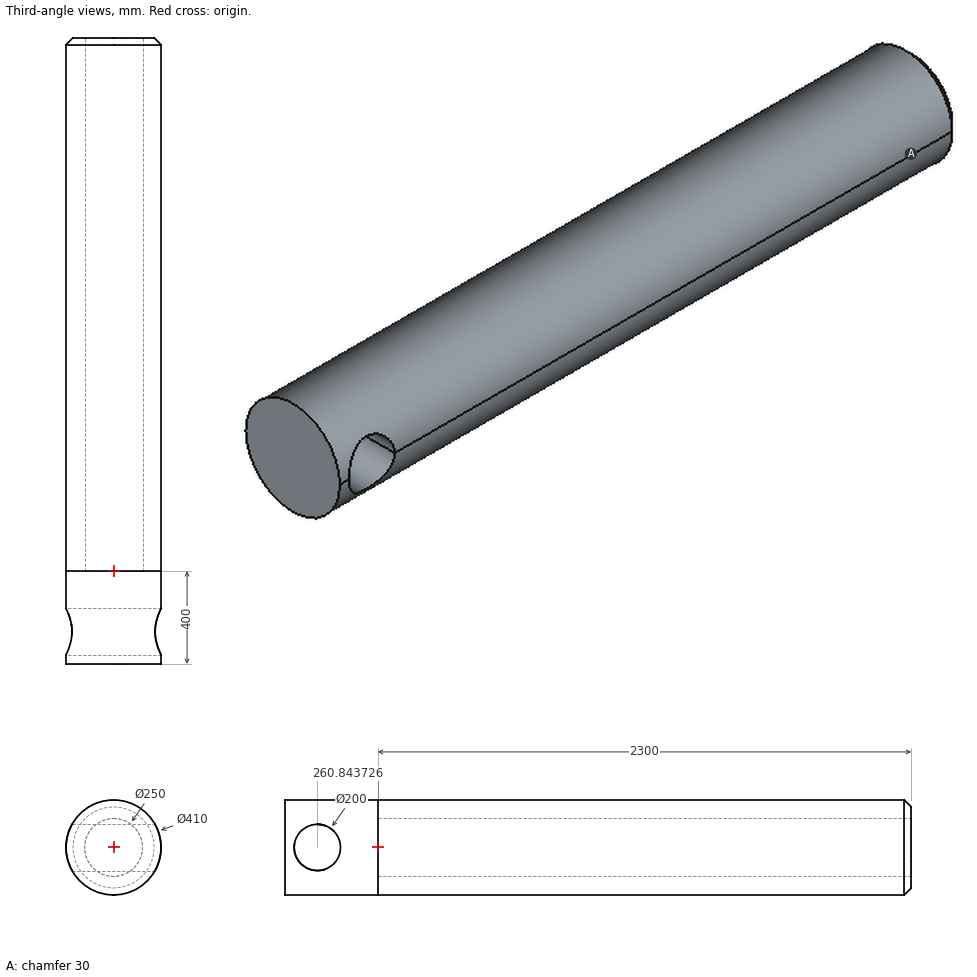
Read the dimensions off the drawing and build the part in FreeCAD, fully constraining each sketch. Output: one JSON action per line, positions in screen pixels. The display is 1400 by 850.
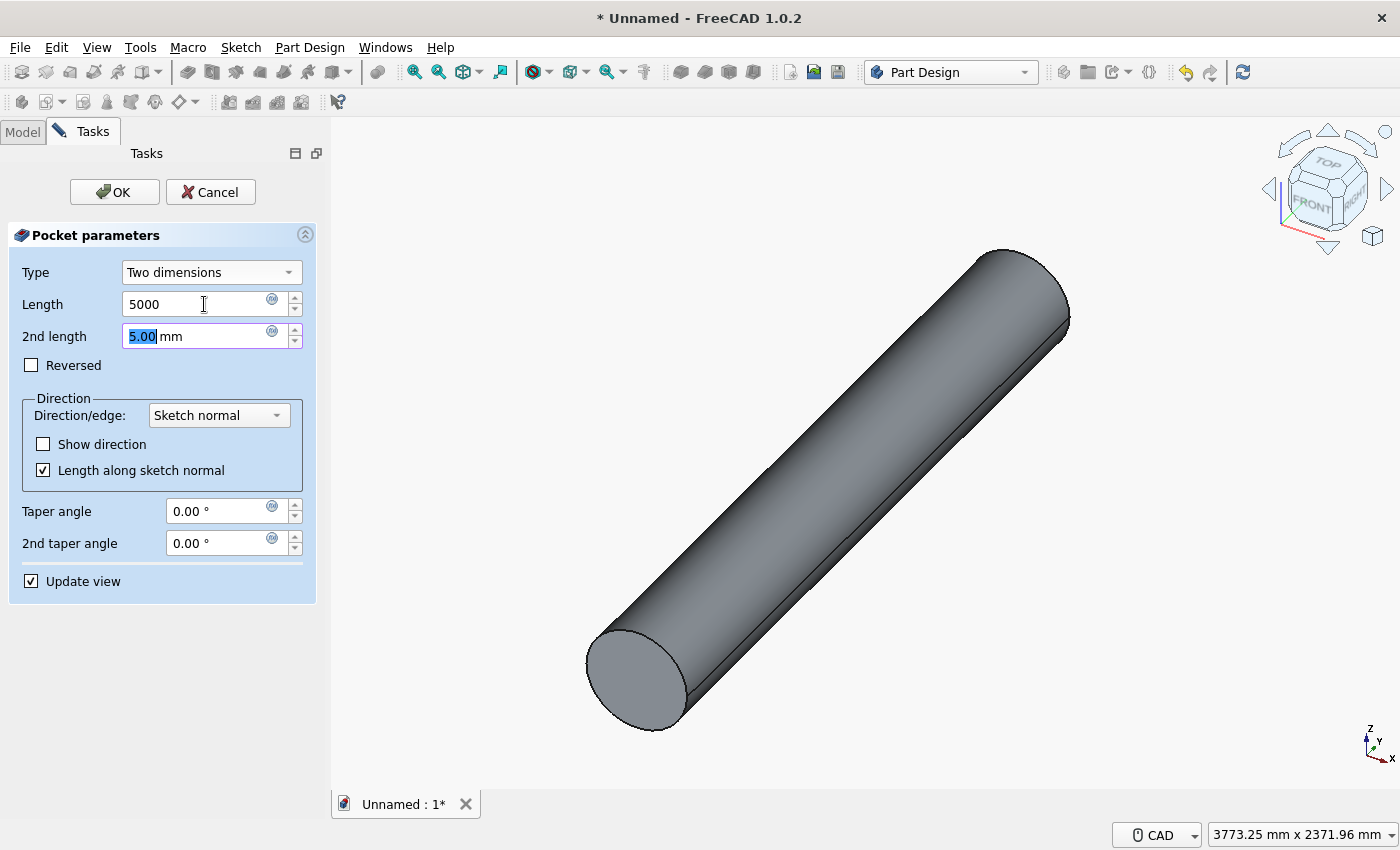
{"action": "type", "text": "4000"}
{"action": "key", "text": "Tab"}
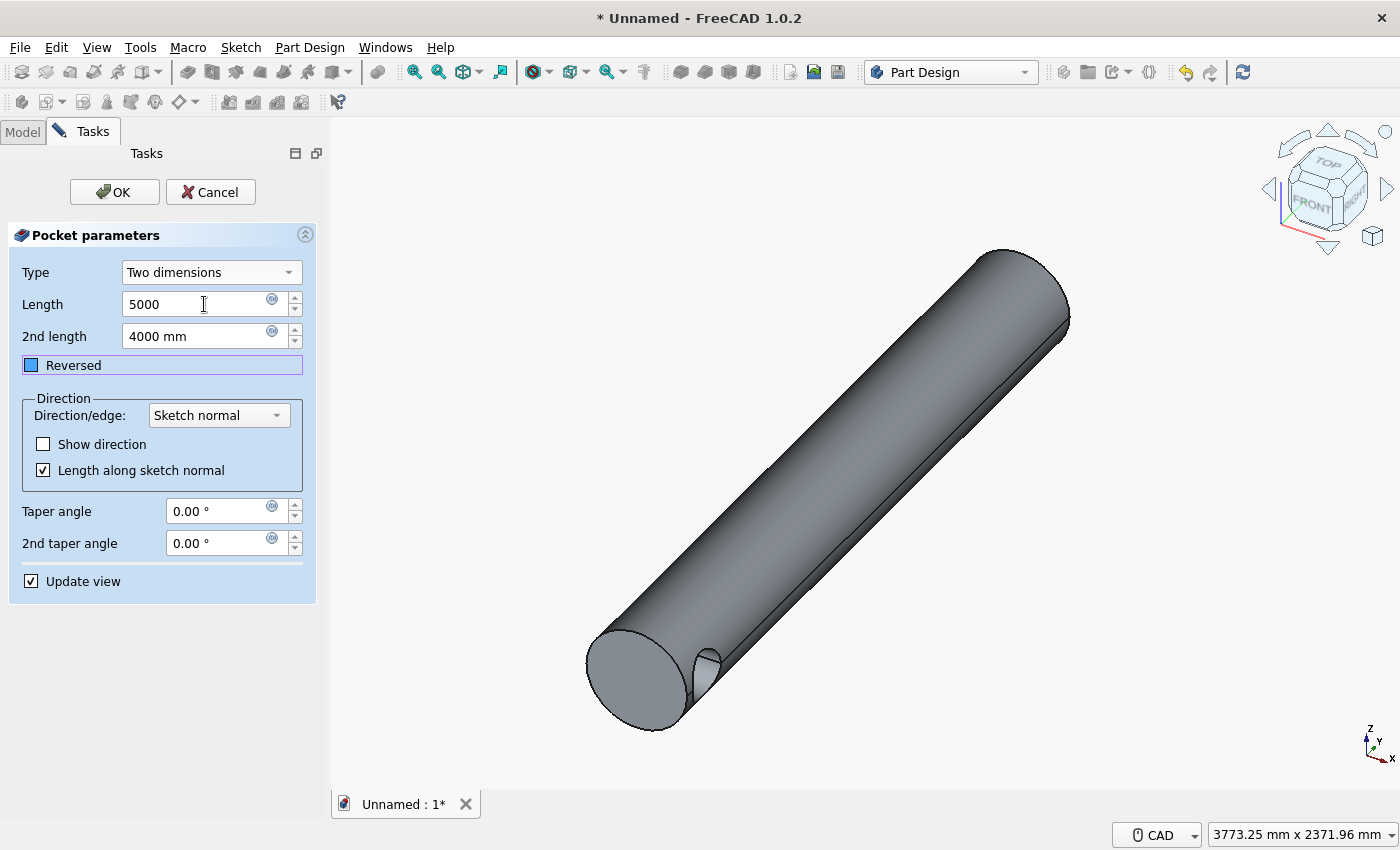
{"action": "left_click", "coordinate": [30, 365]}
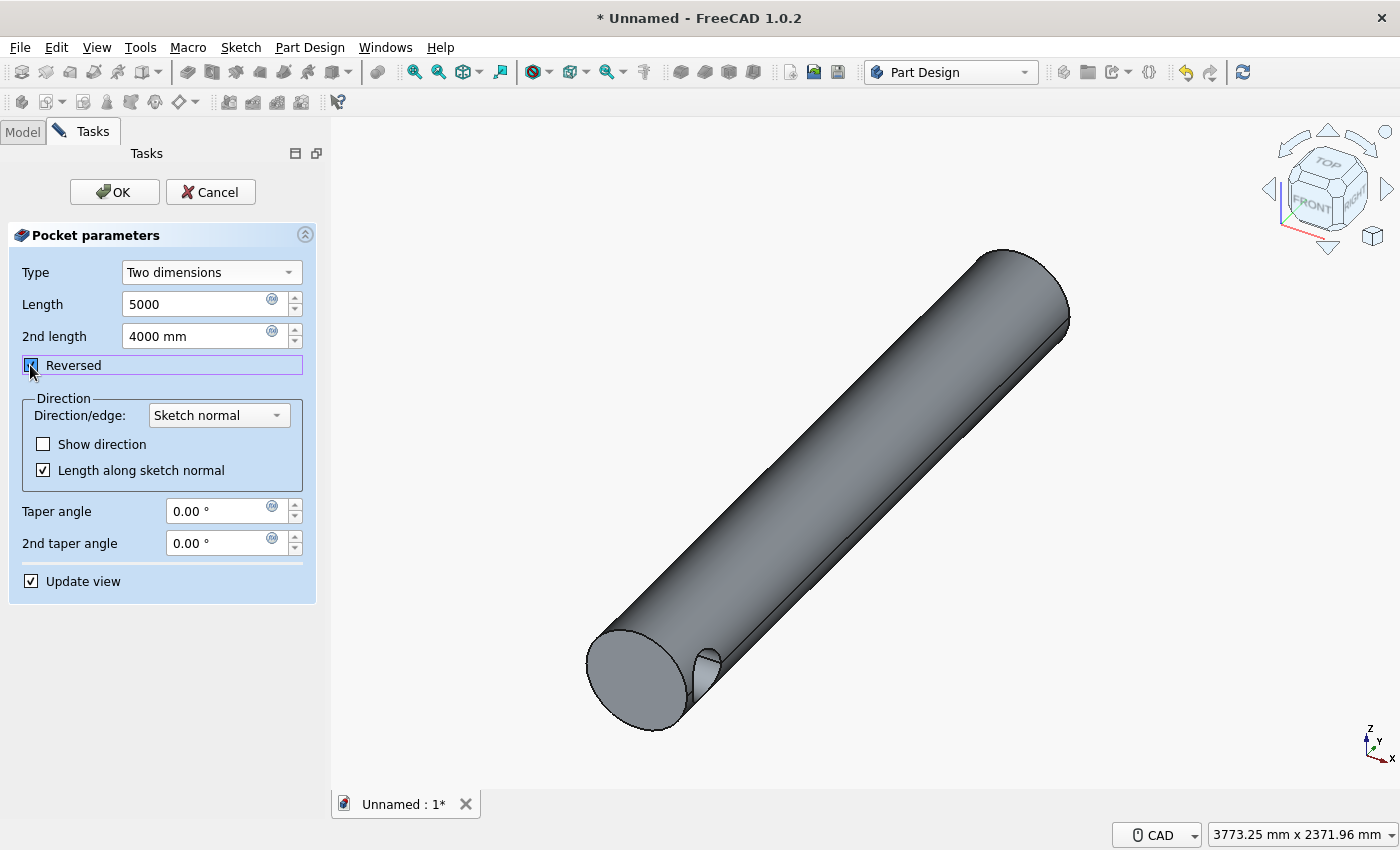
{"action": "left_click", "coordinate": [115, 192]}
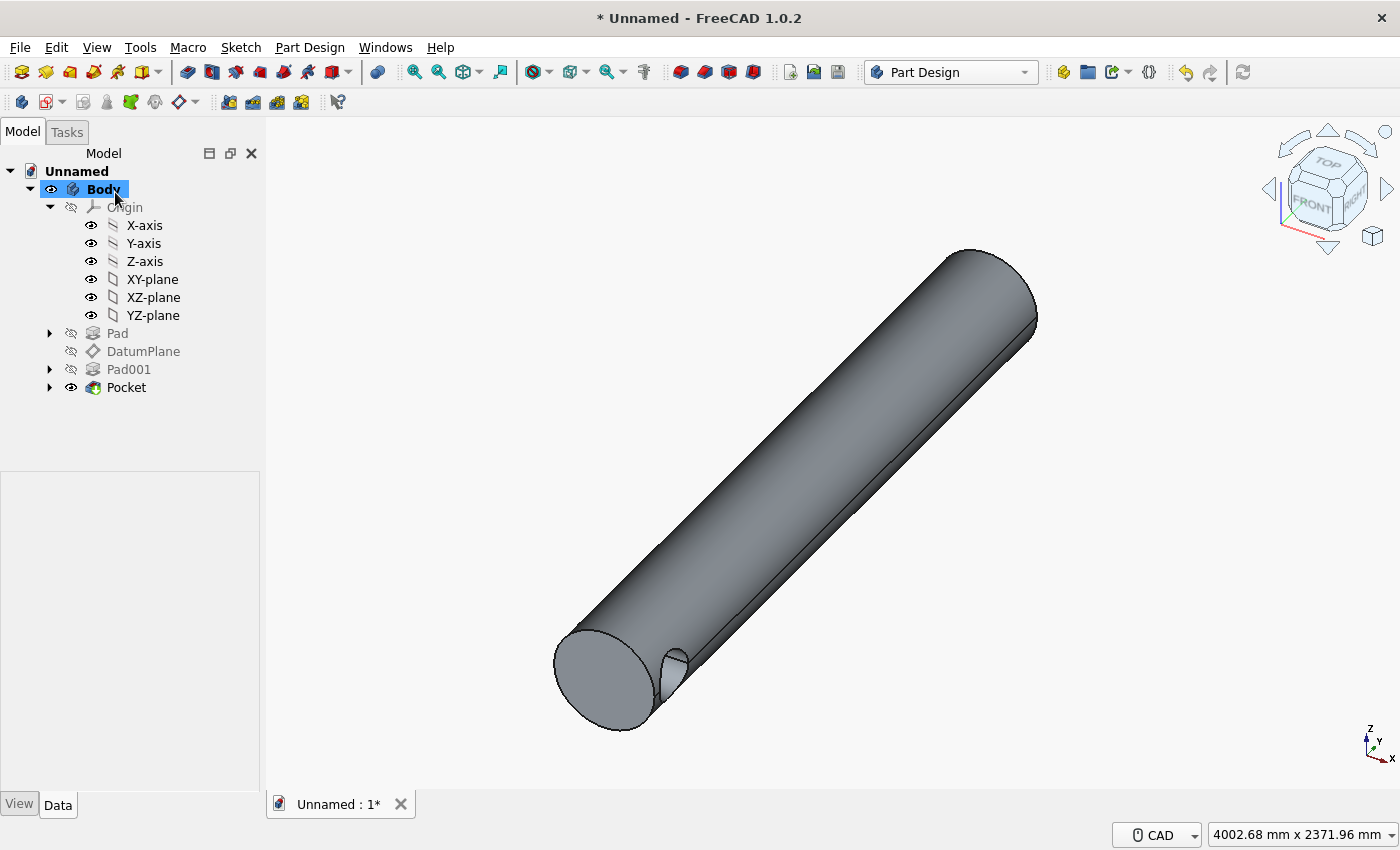
{"action": "key", "text": "0"}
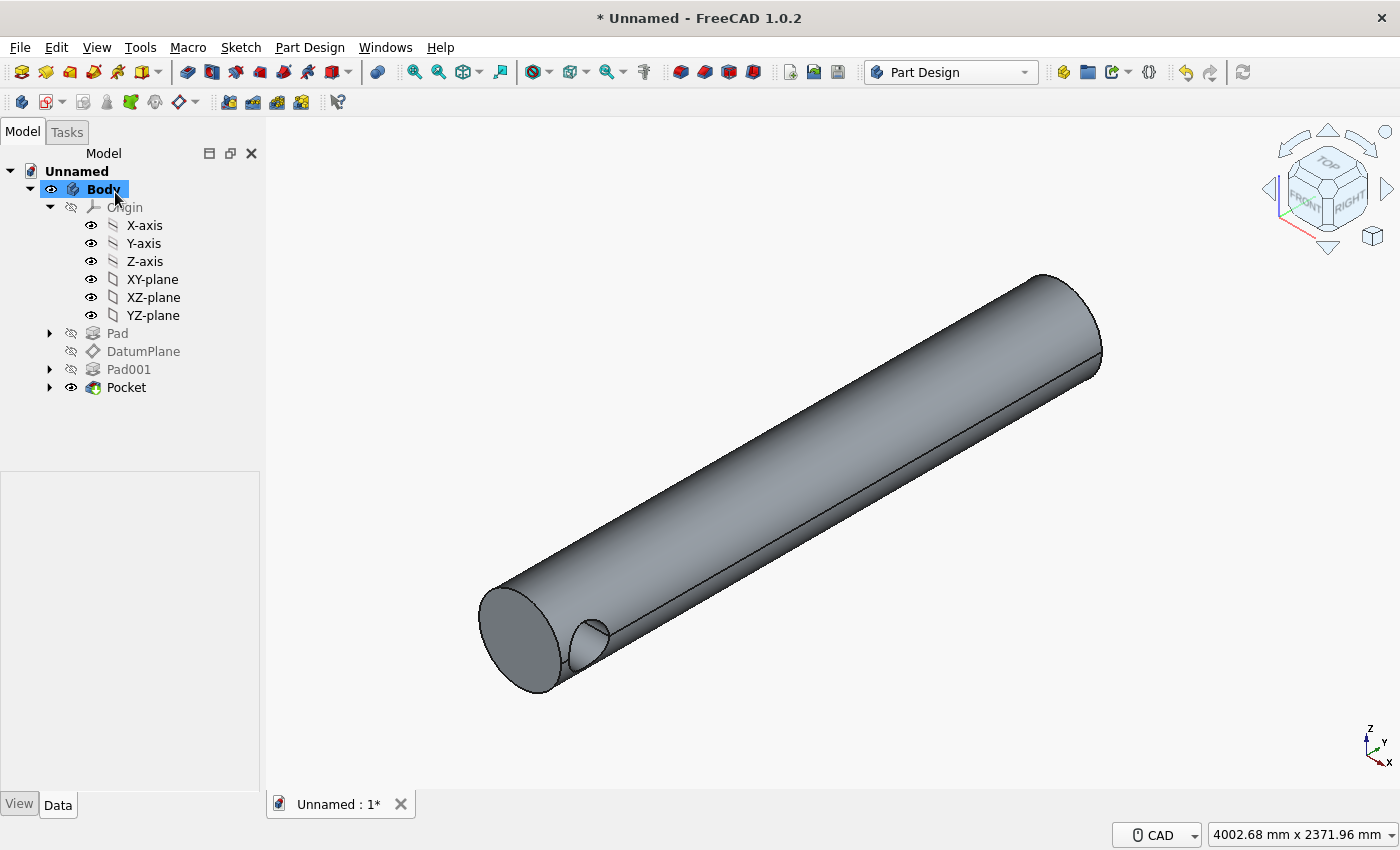
{"action": "key", "text": "2"}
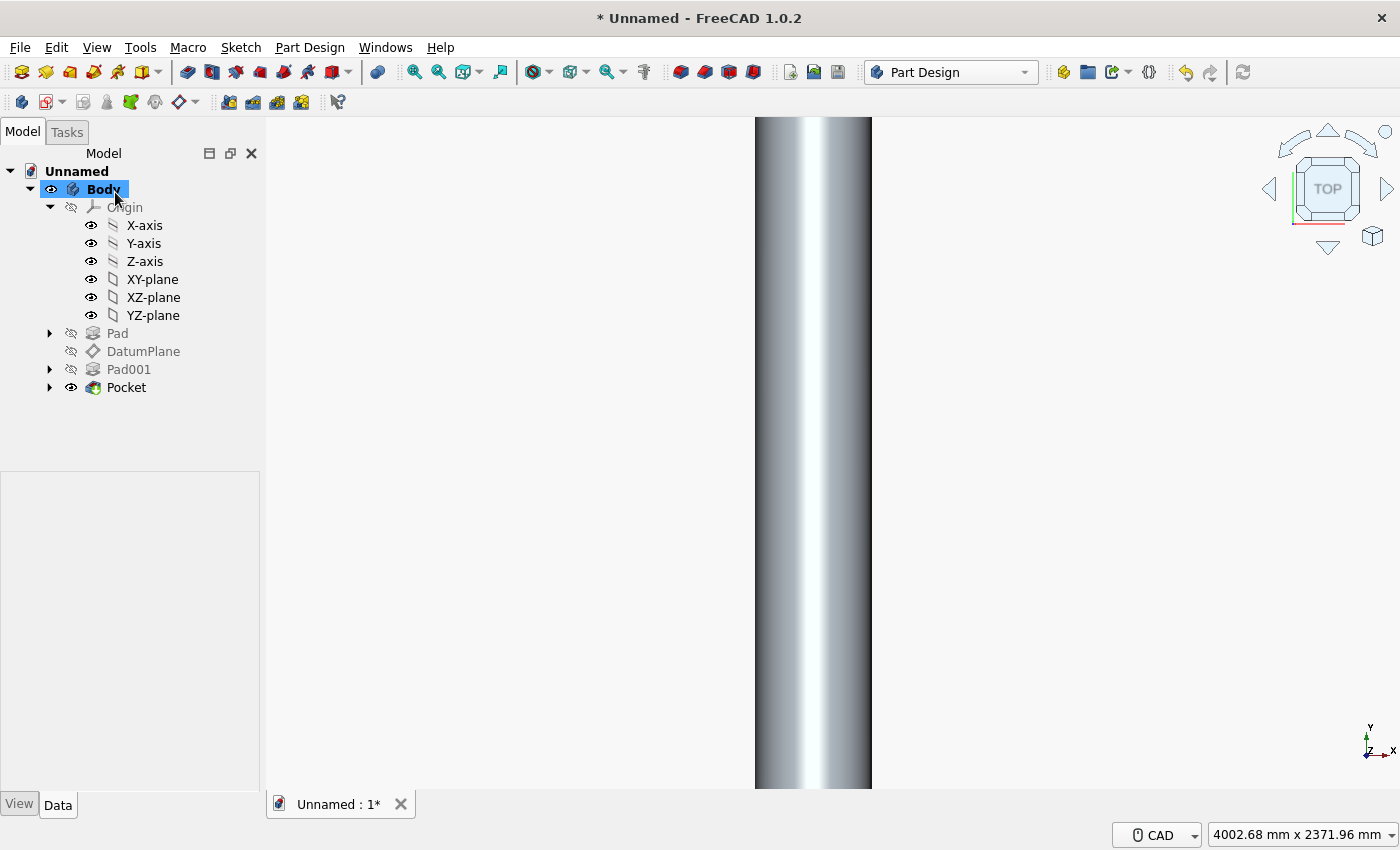
{"action": "left_click", "coordinate": [416, 72]}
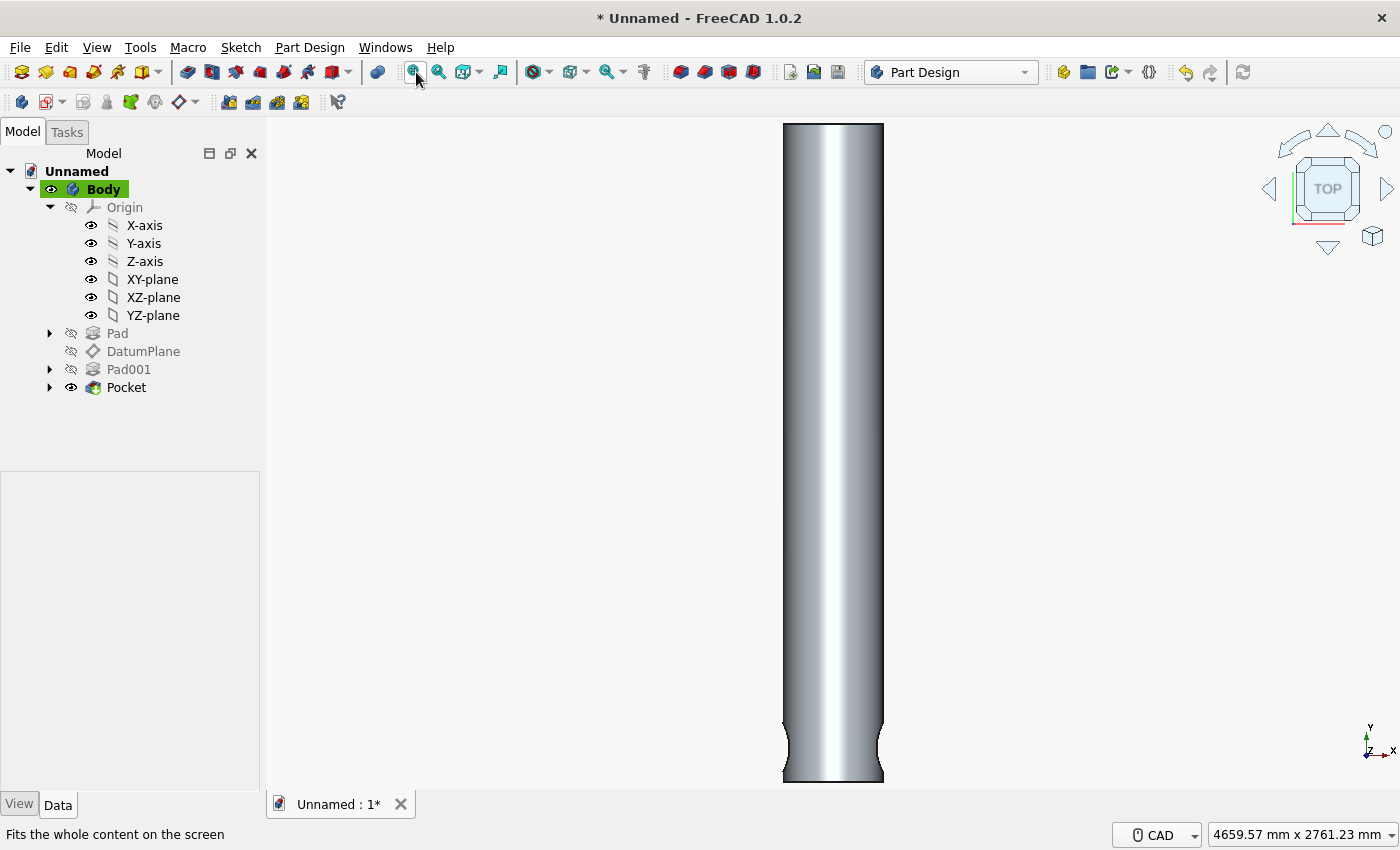
{"action": "key", "text": "1"}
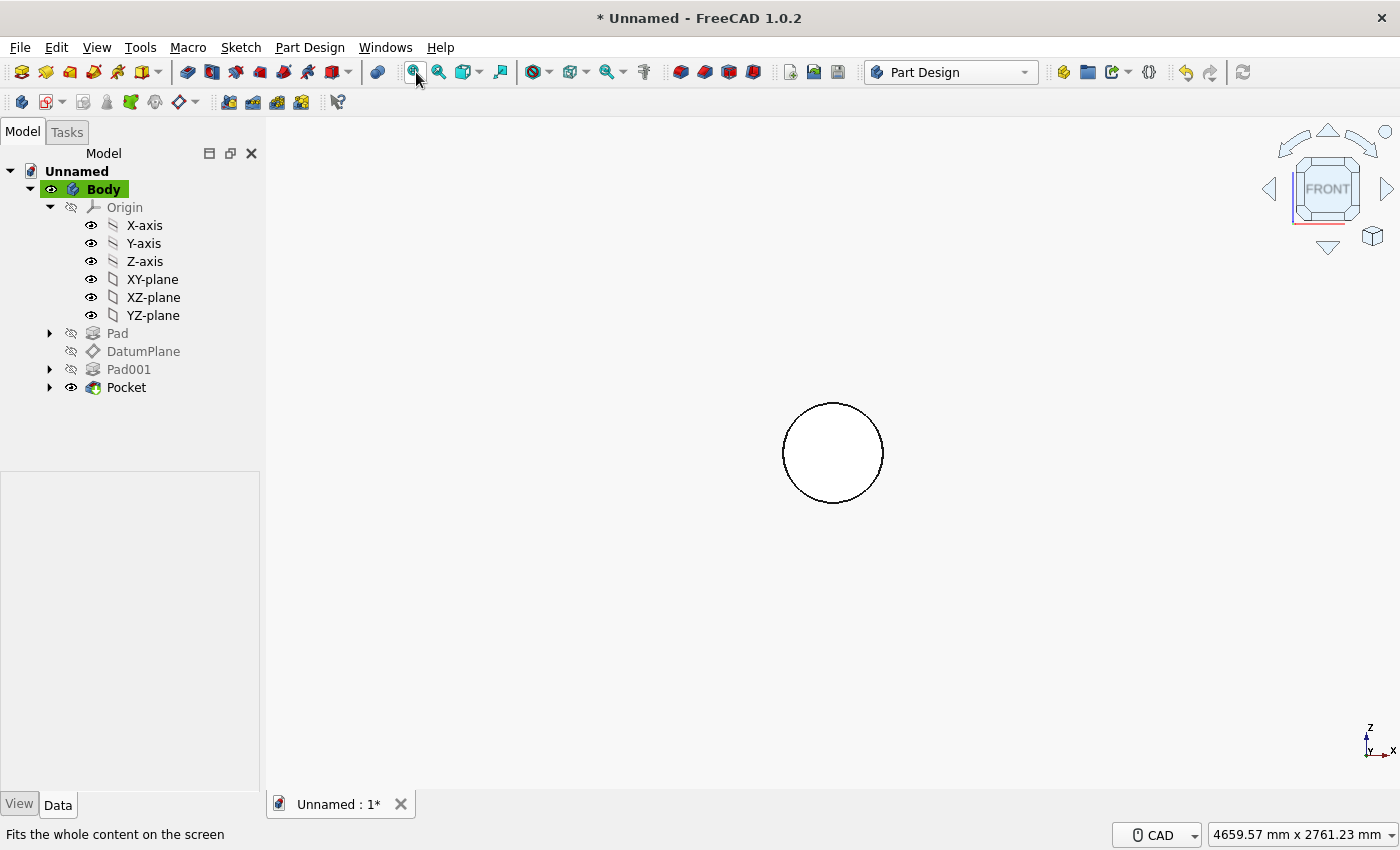
{"action": "left_click", "coordinate": [416, 72]}